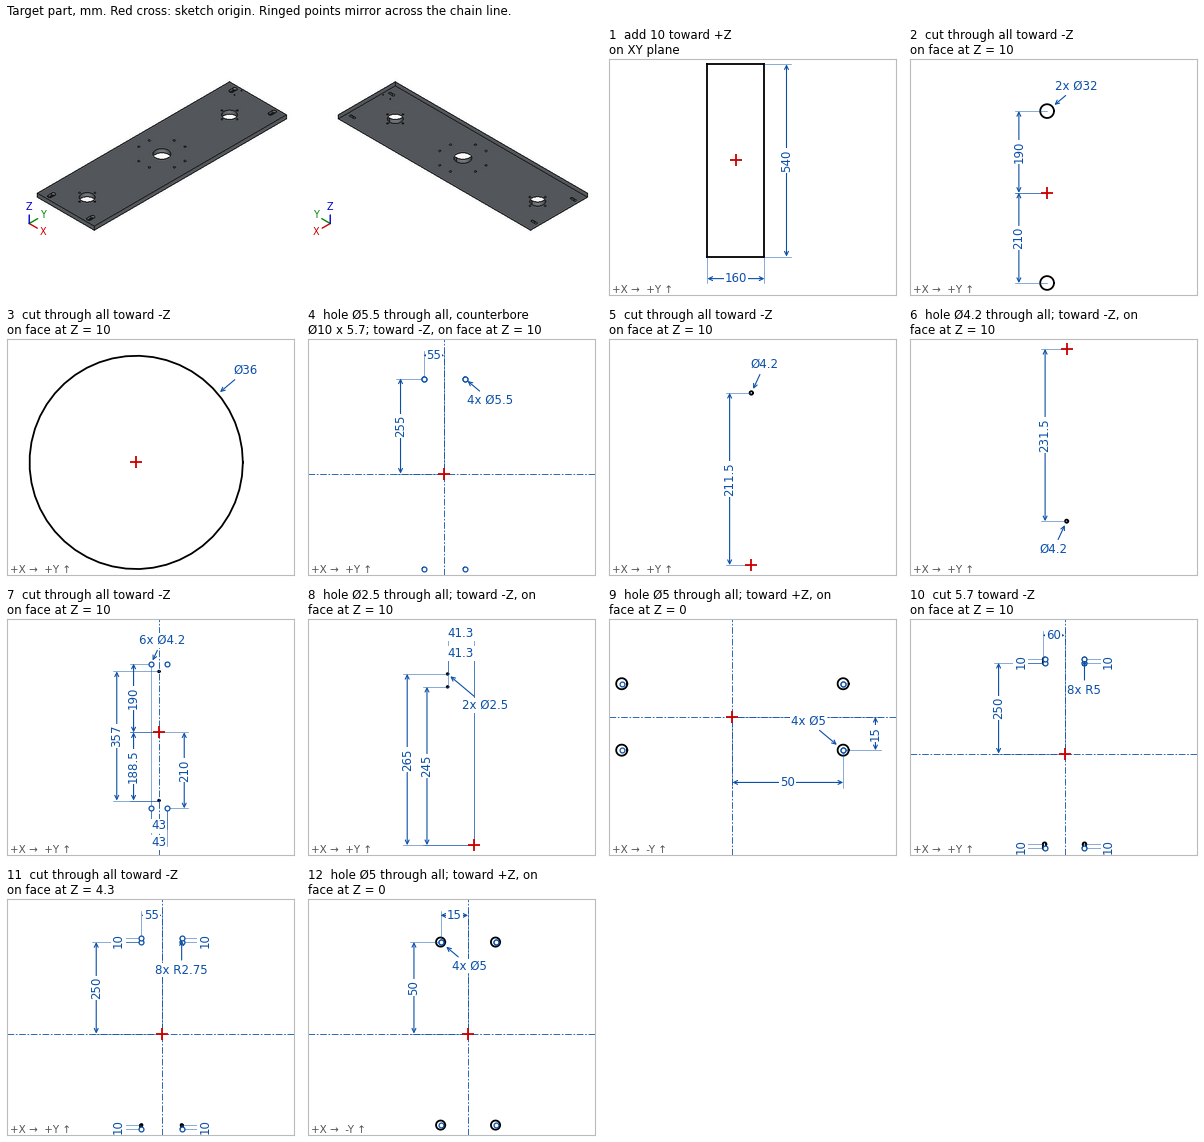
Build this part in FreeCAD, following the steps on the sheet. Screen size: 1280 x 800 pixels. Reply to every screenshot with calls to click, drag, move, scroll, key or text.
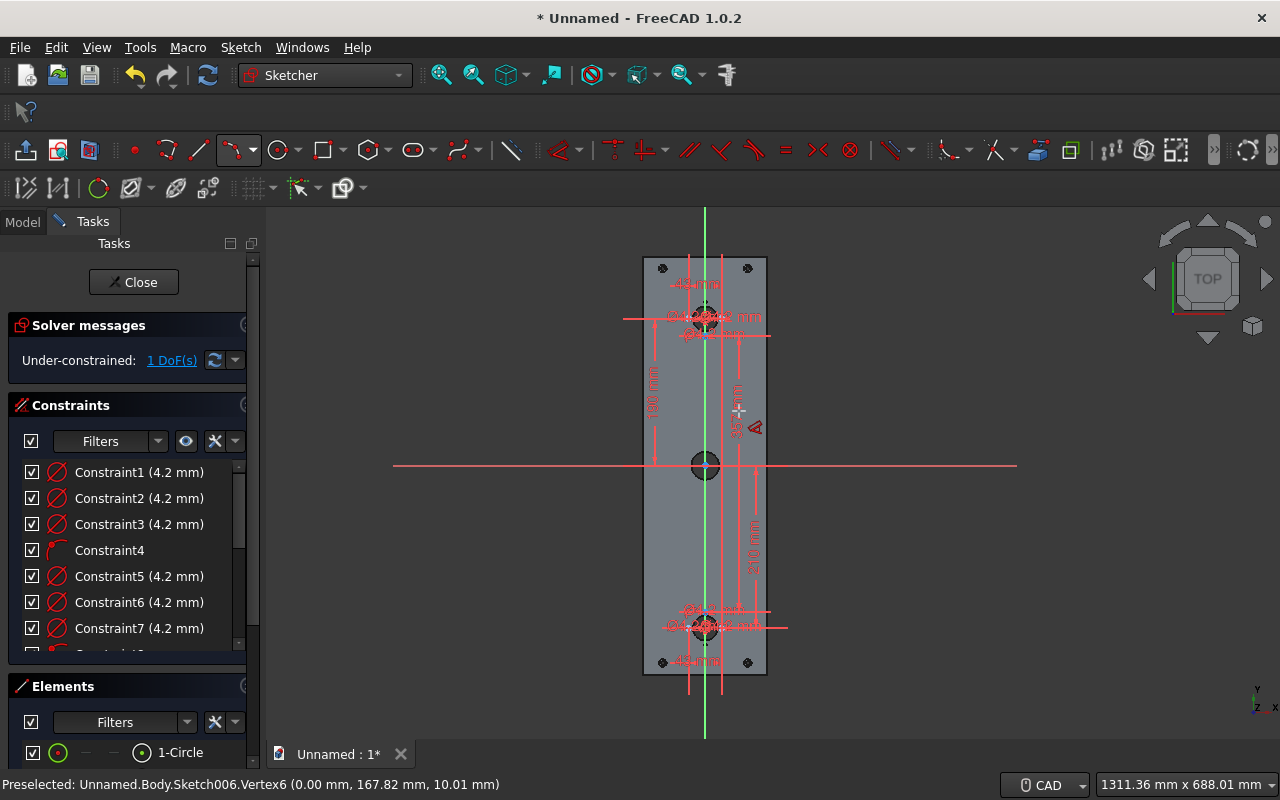
click(705, 612)
click(739, 505)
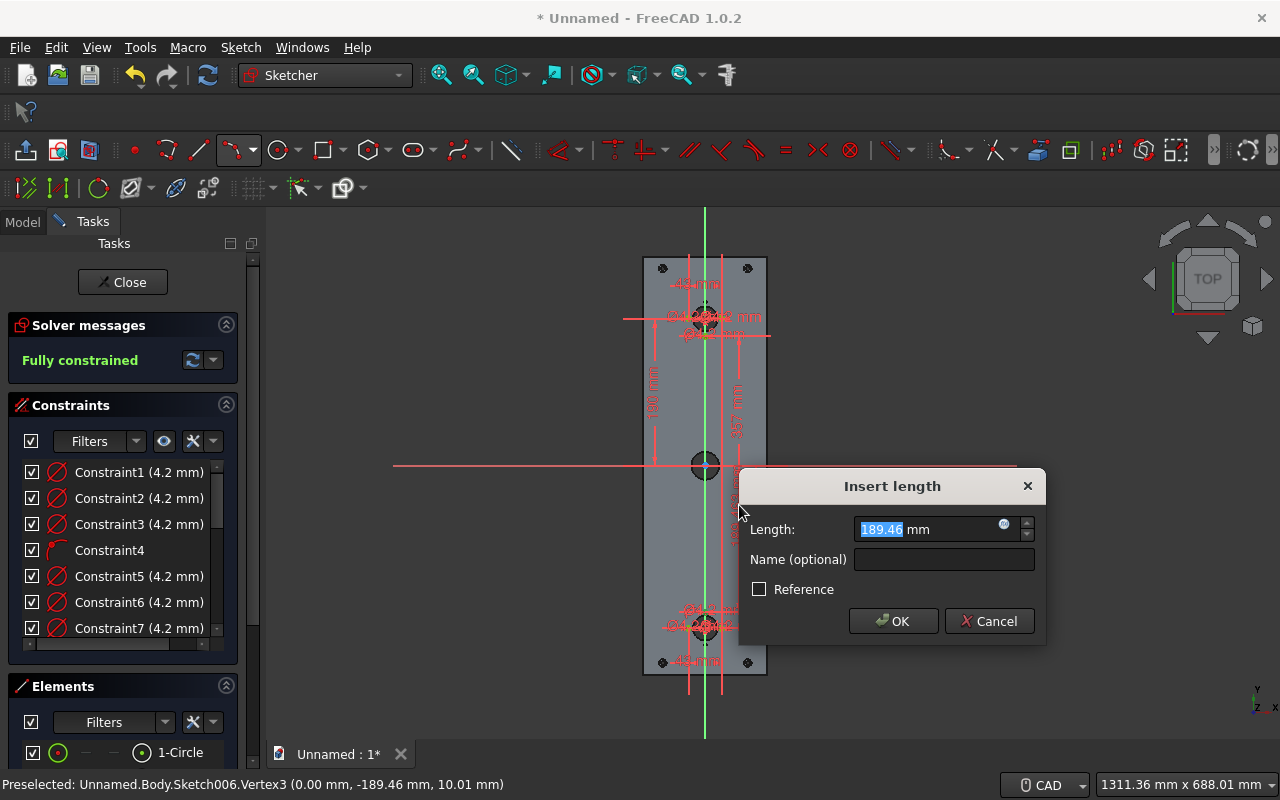
text(188.5)
key(Return)
key(Escape)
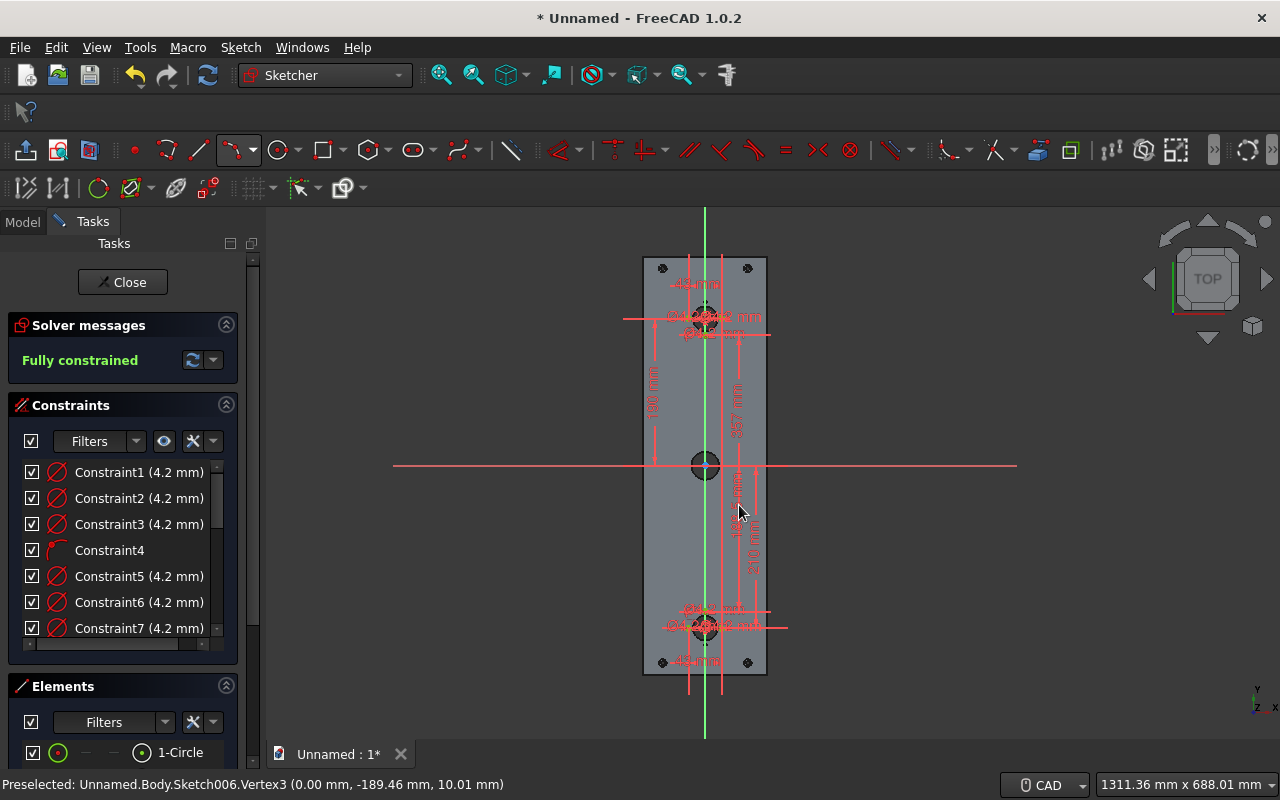
click(123, 282)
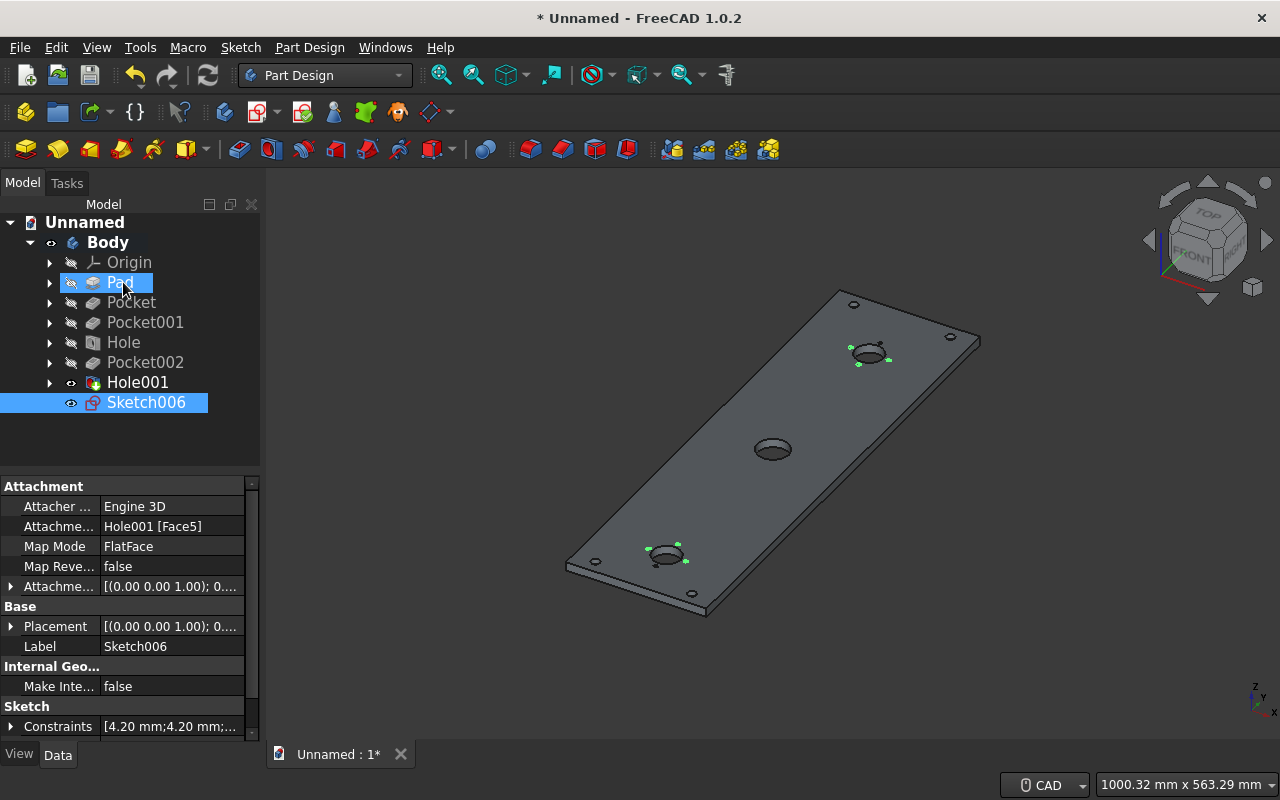
click(240, 150)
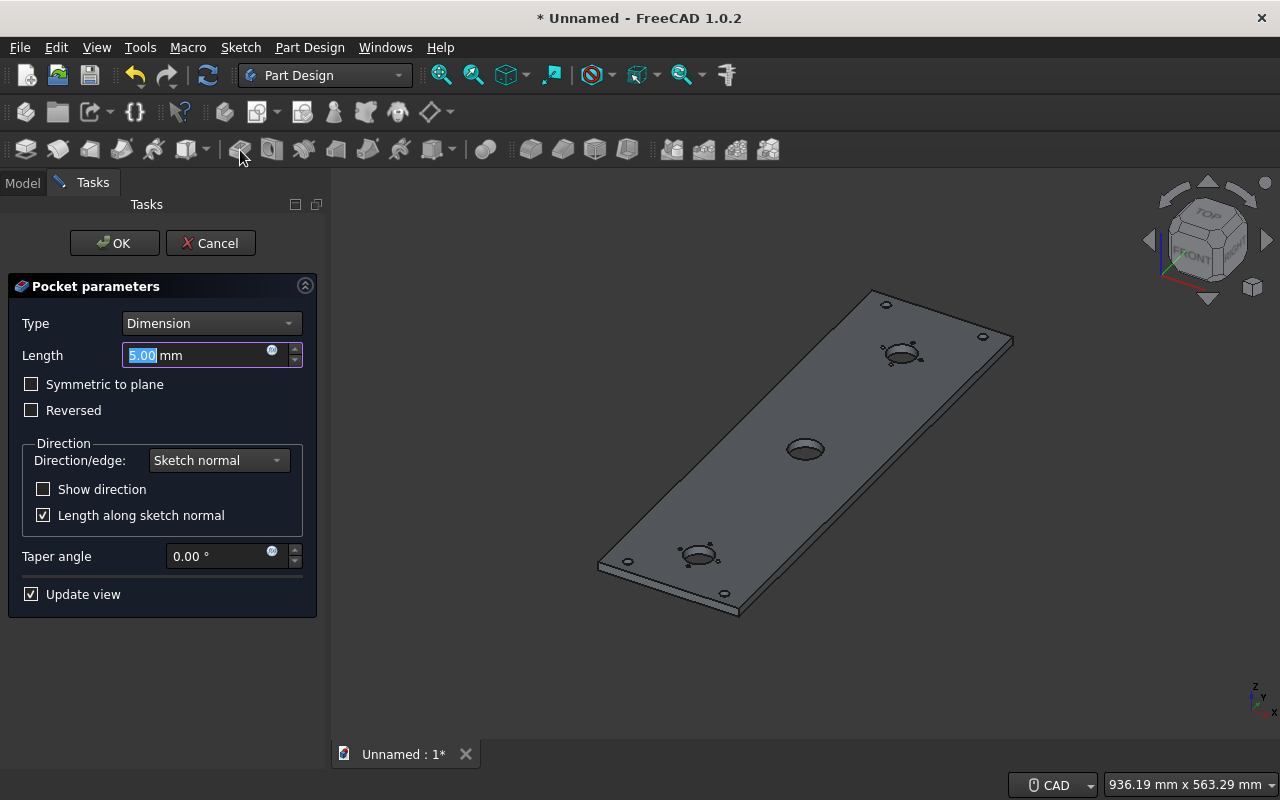
click(212, 324)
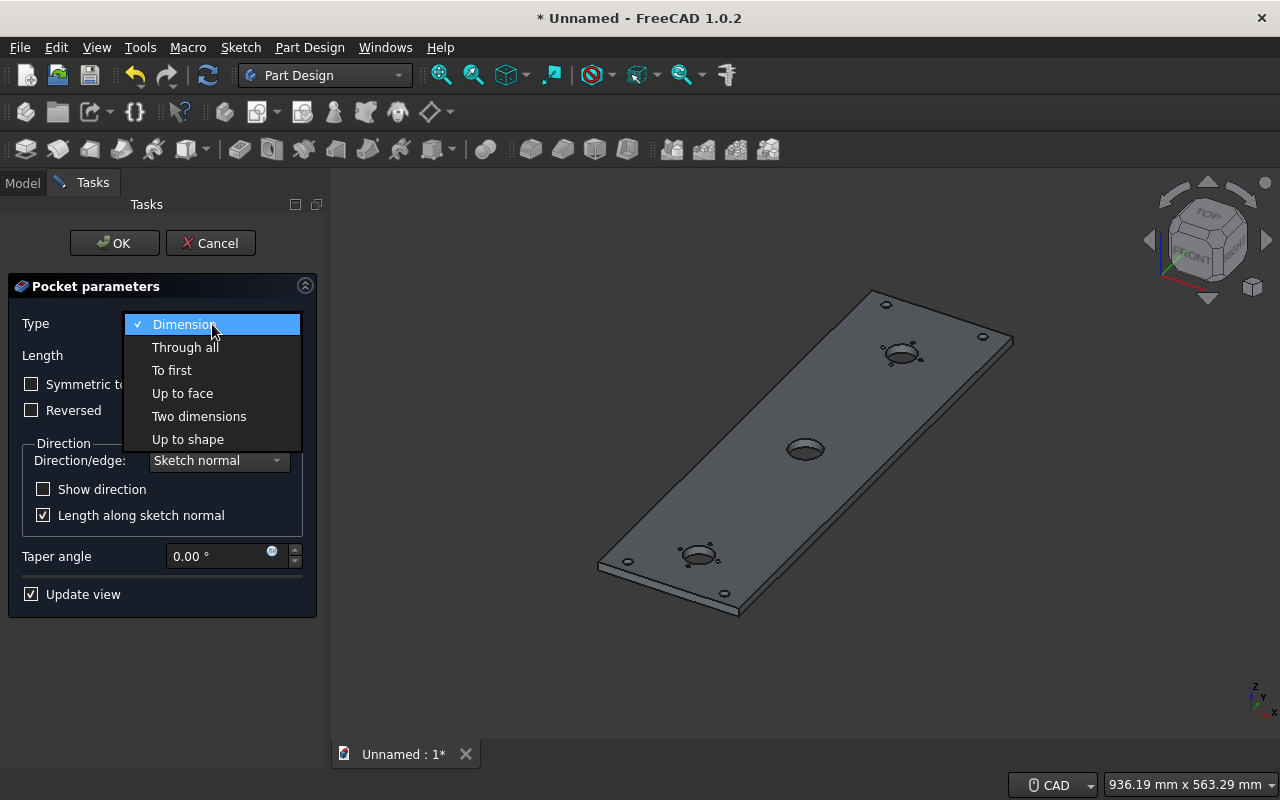
click(212, 348)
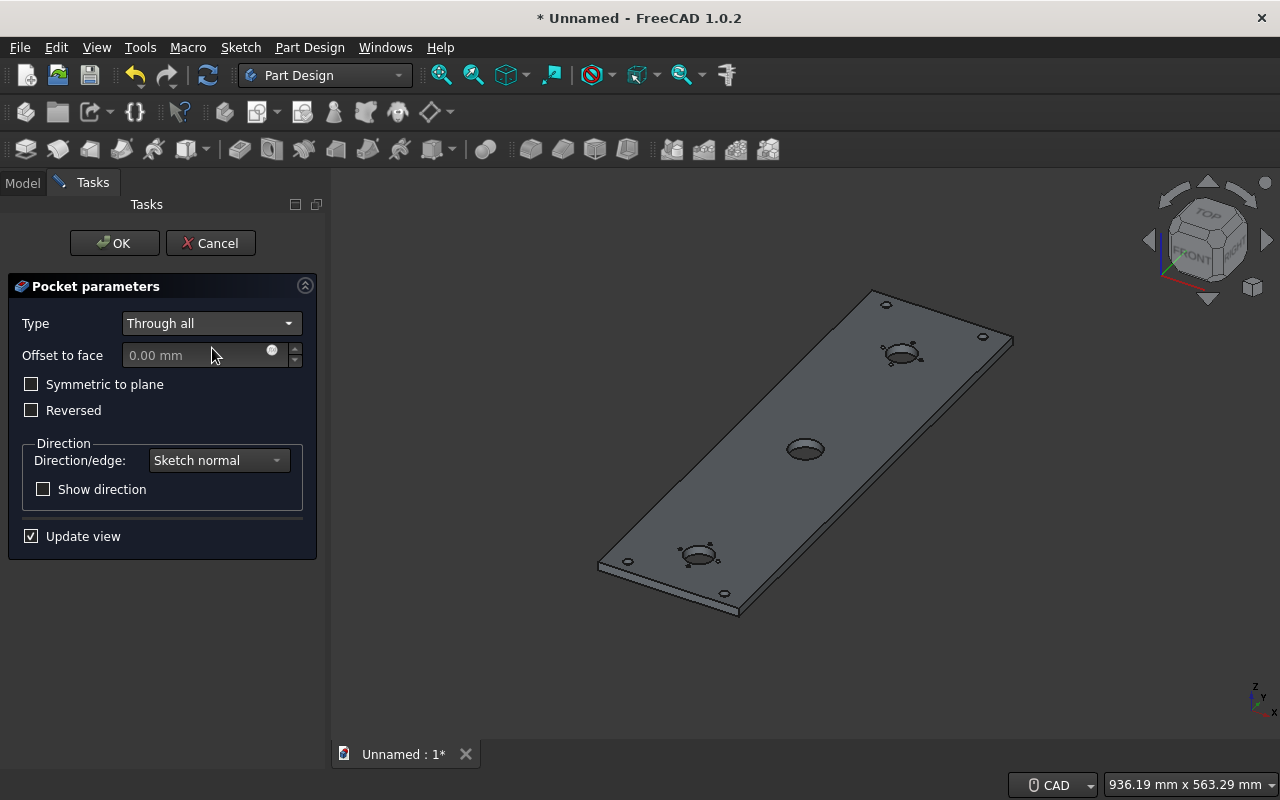
click(115, 243)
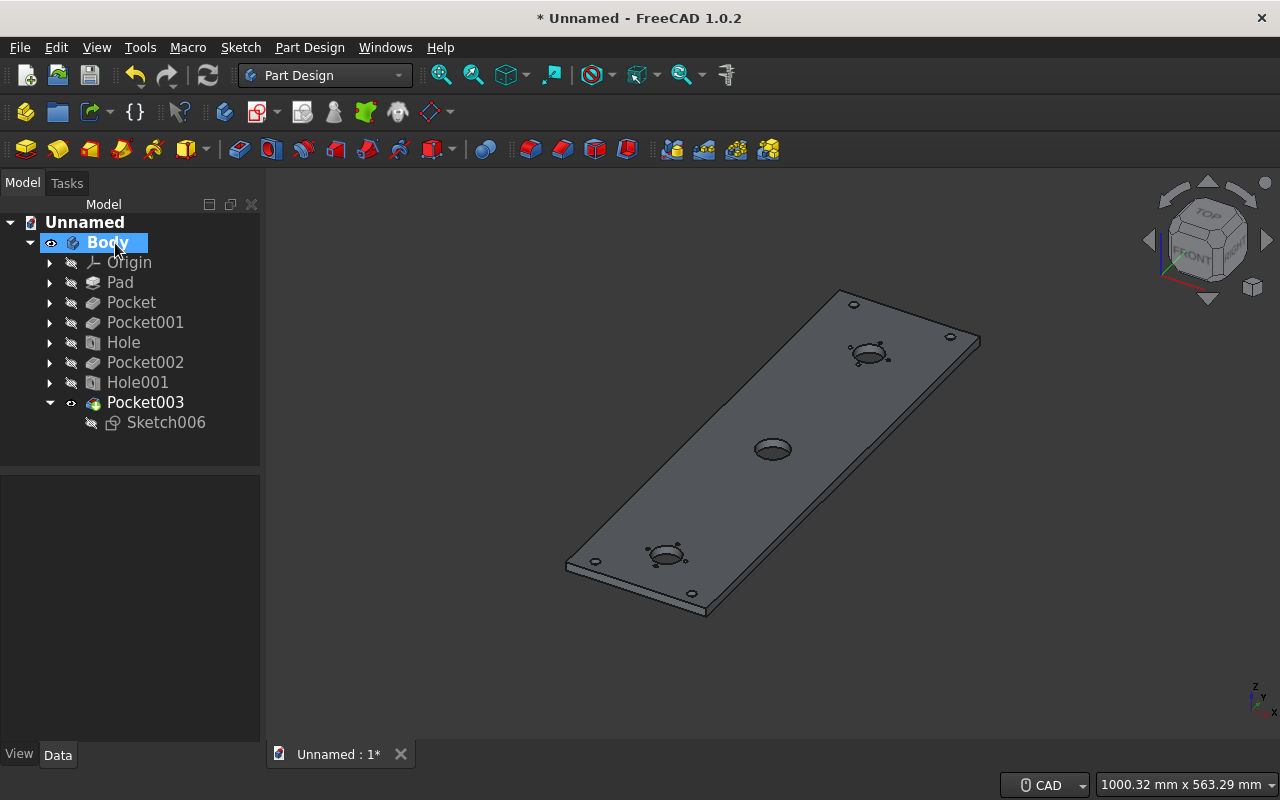
click(812, 410)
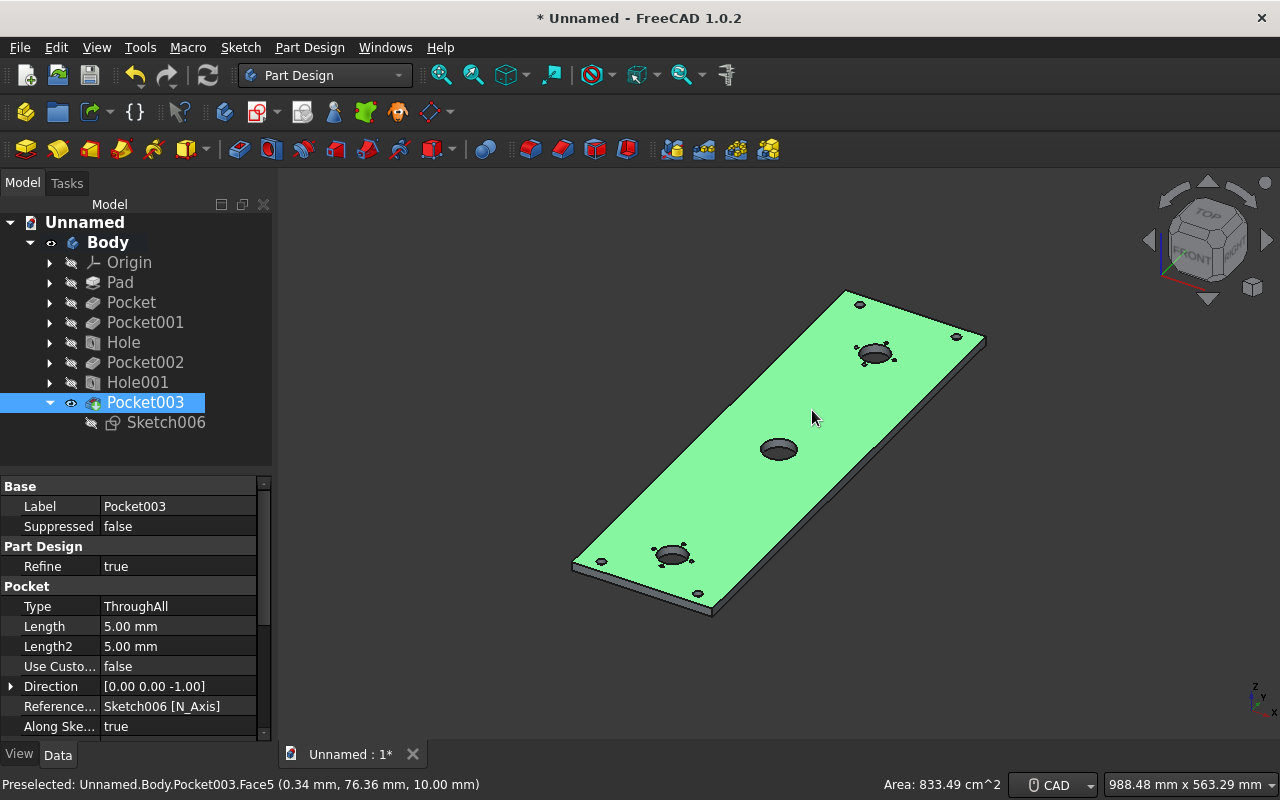
click(258, 112)